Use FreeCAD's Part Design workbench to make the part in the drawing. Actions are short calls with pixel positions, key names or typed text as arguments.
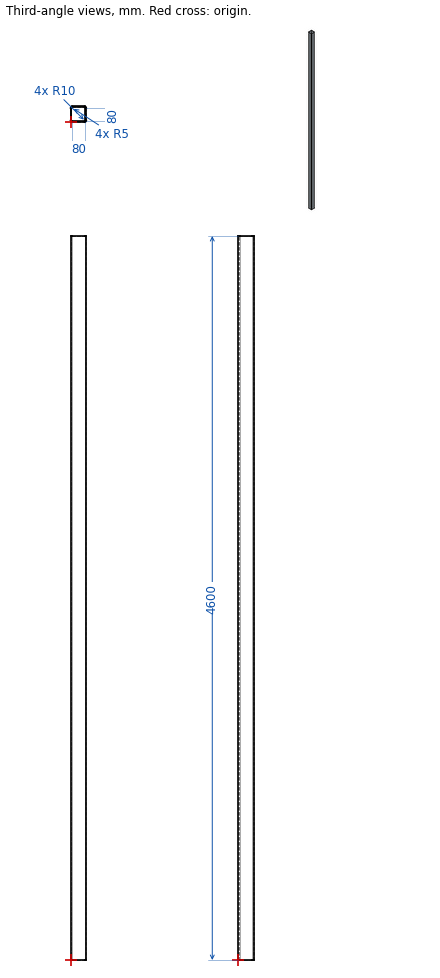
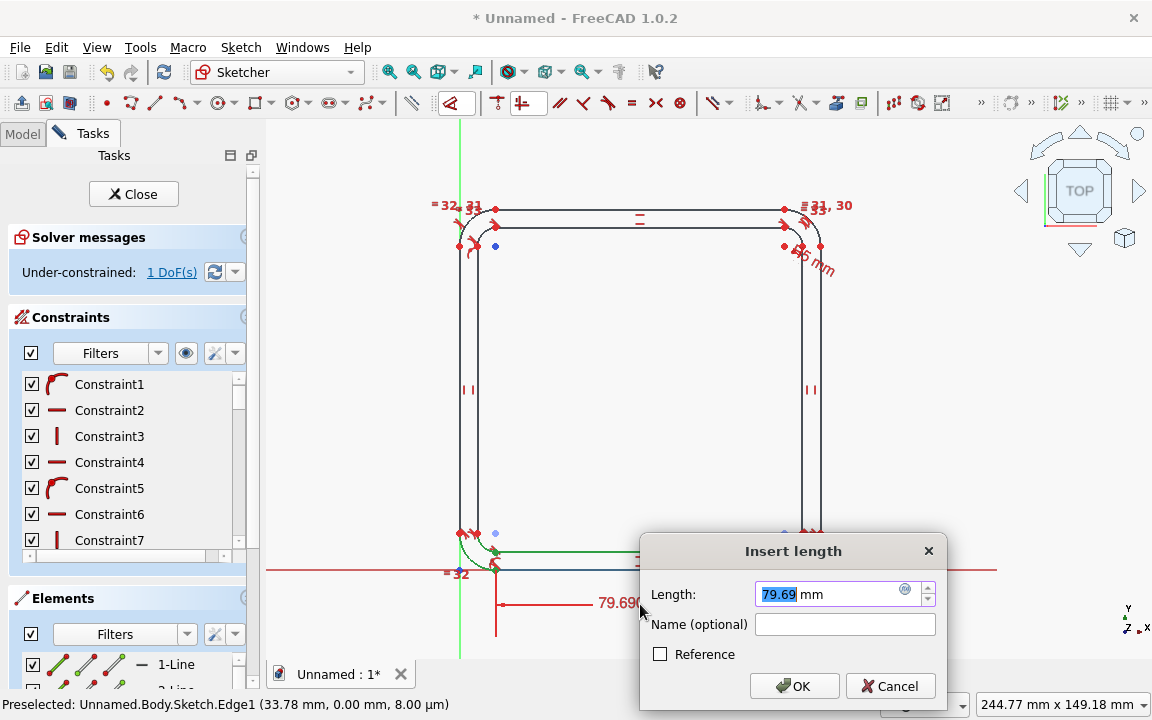
text(80)
key(Return)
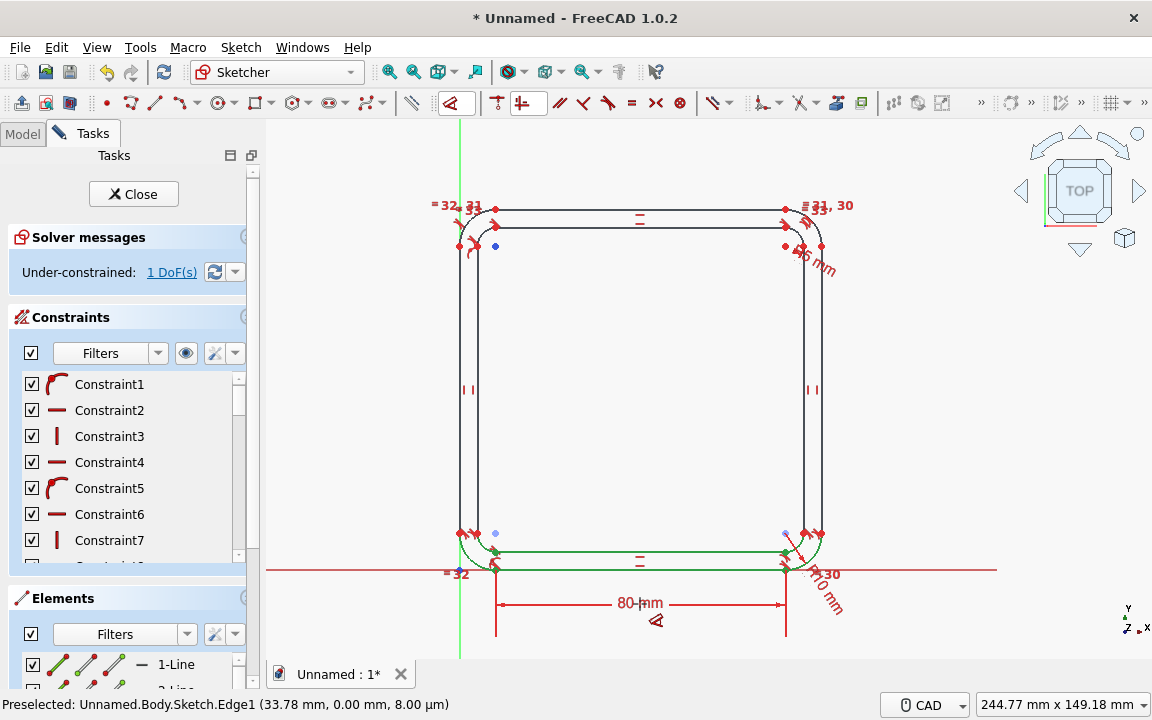
click(822, 448)
click(856, 390)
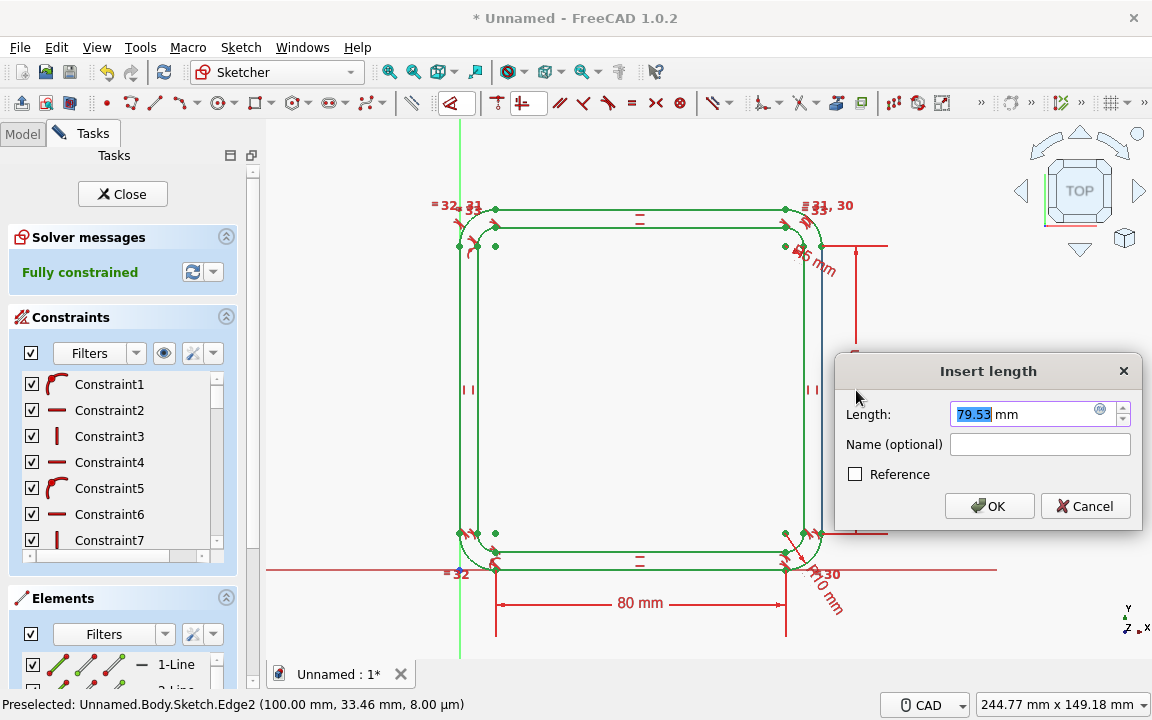
text(80)
key(Return)
key(Escape)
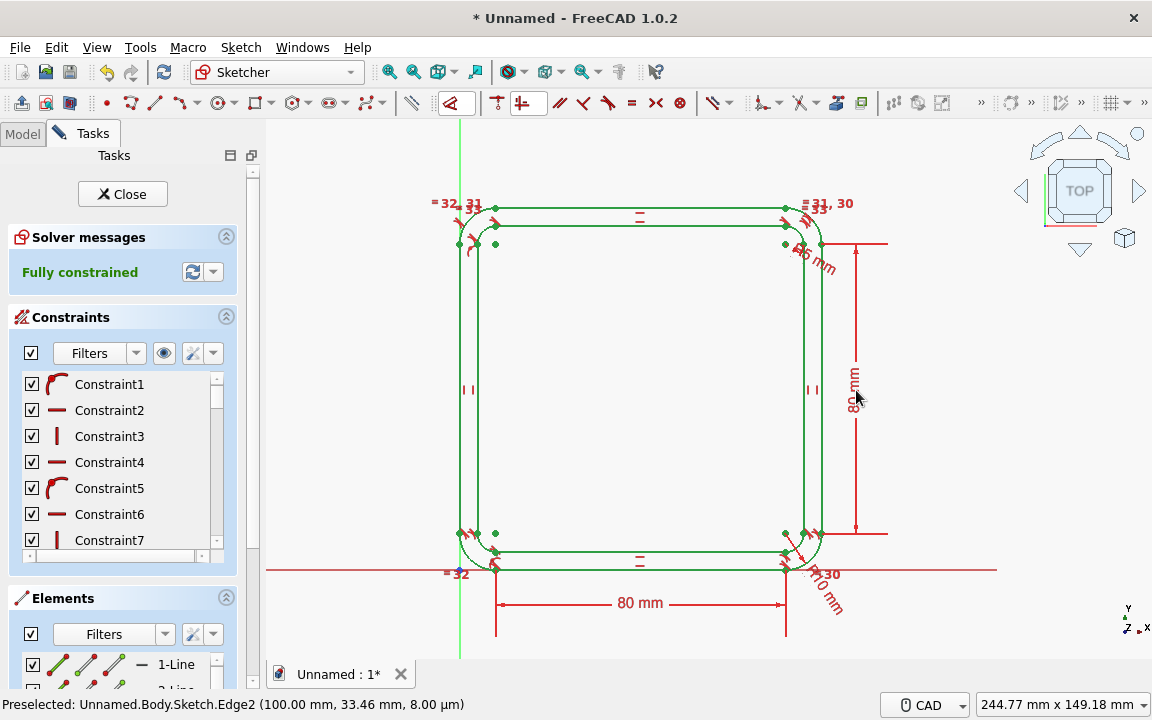
click(123, 194)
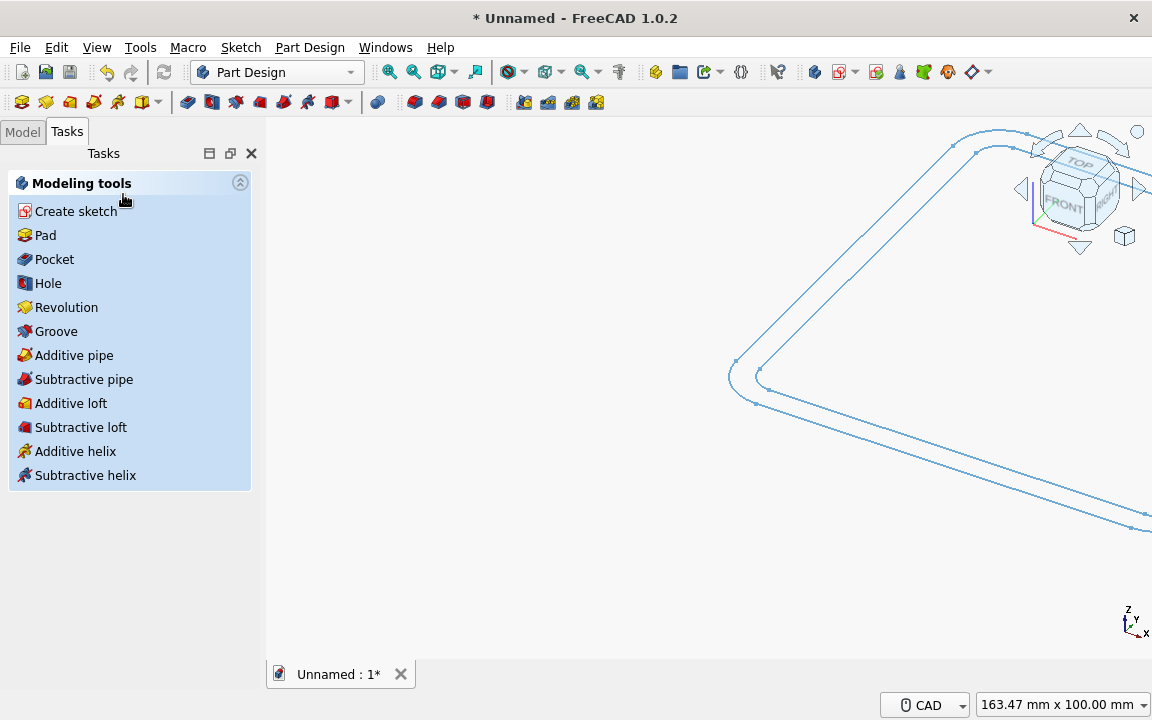
click(22, 102)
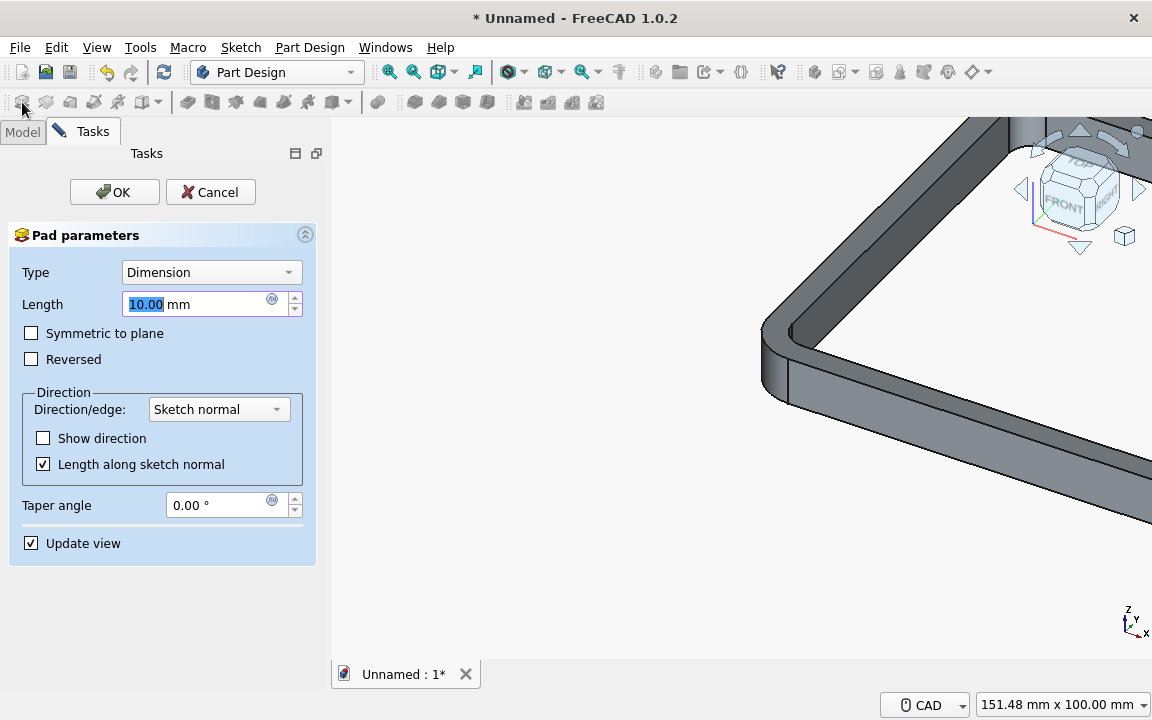
text(4600)
key(Tab)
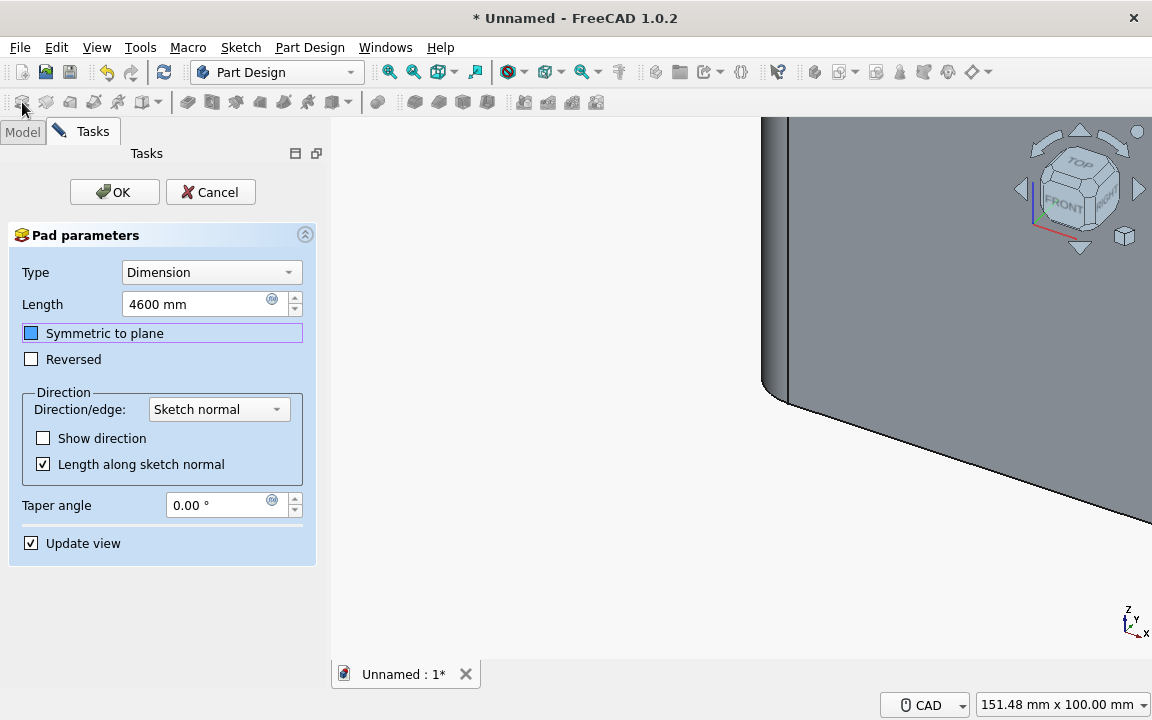
click(115, 192)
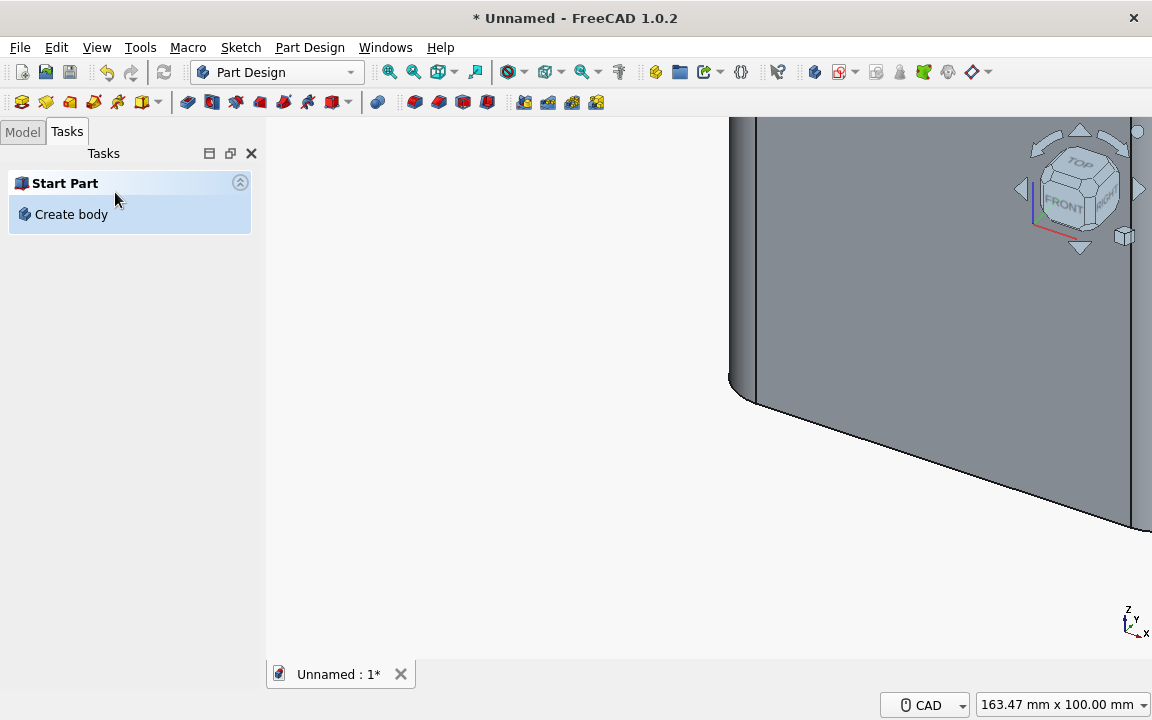
key(0)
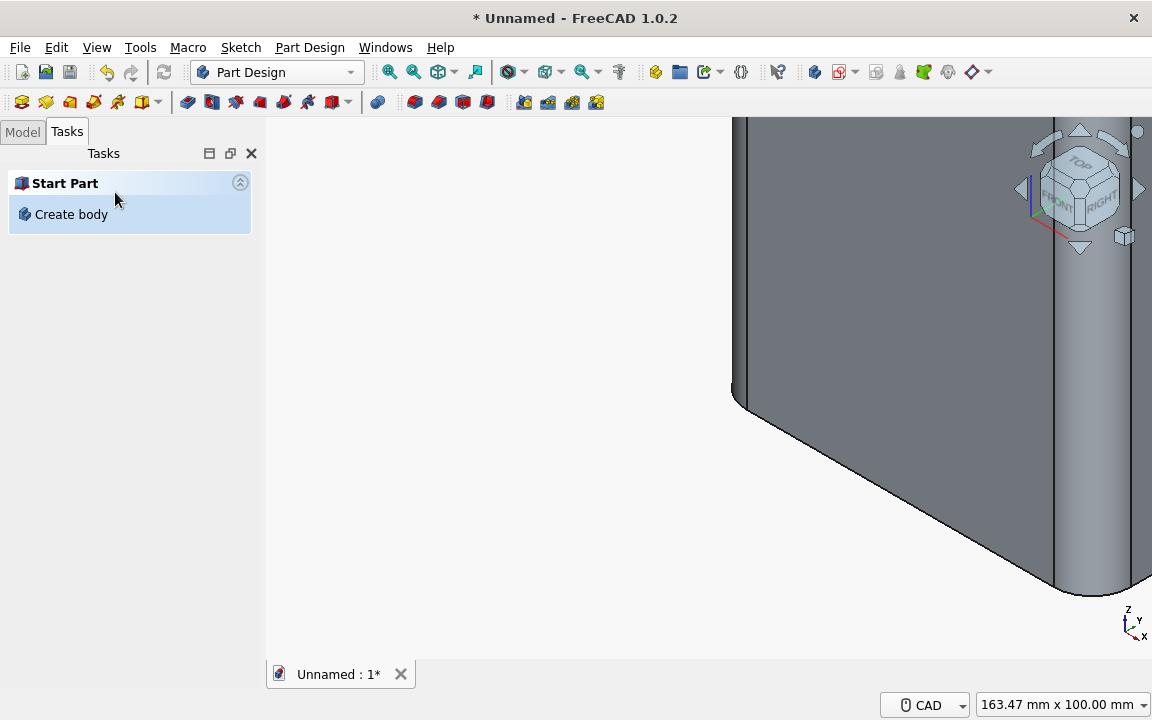
click(390, 72)